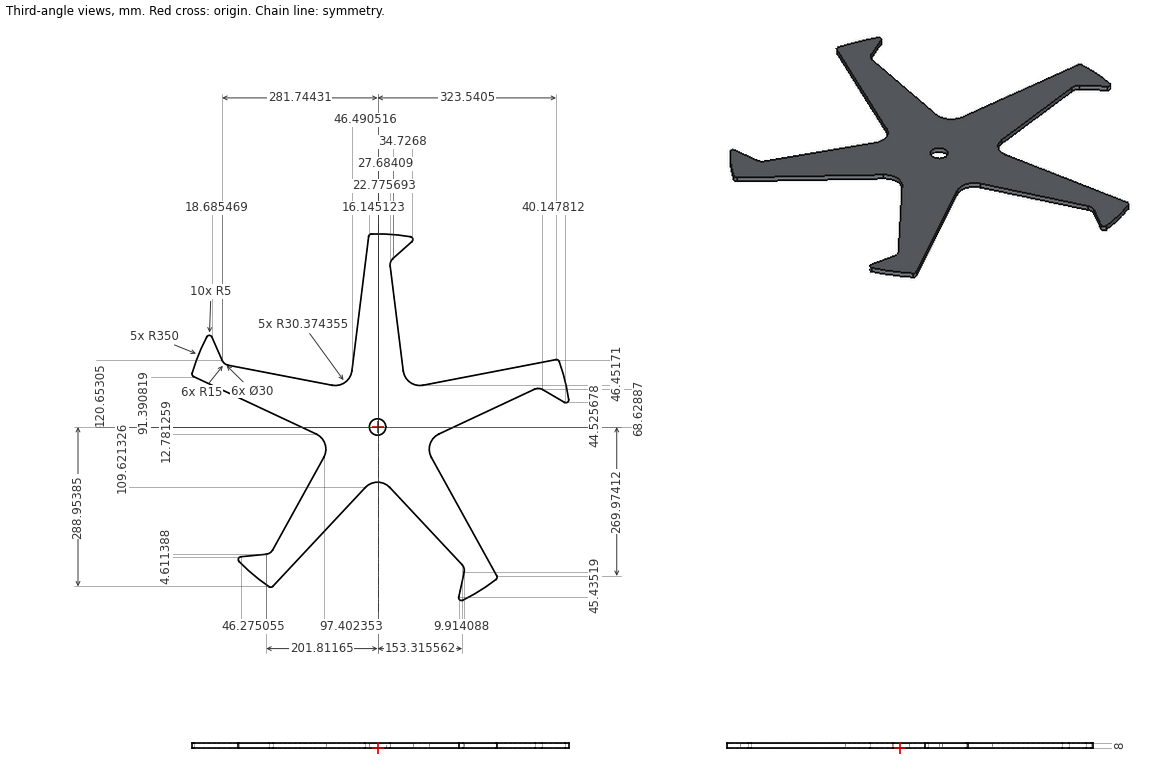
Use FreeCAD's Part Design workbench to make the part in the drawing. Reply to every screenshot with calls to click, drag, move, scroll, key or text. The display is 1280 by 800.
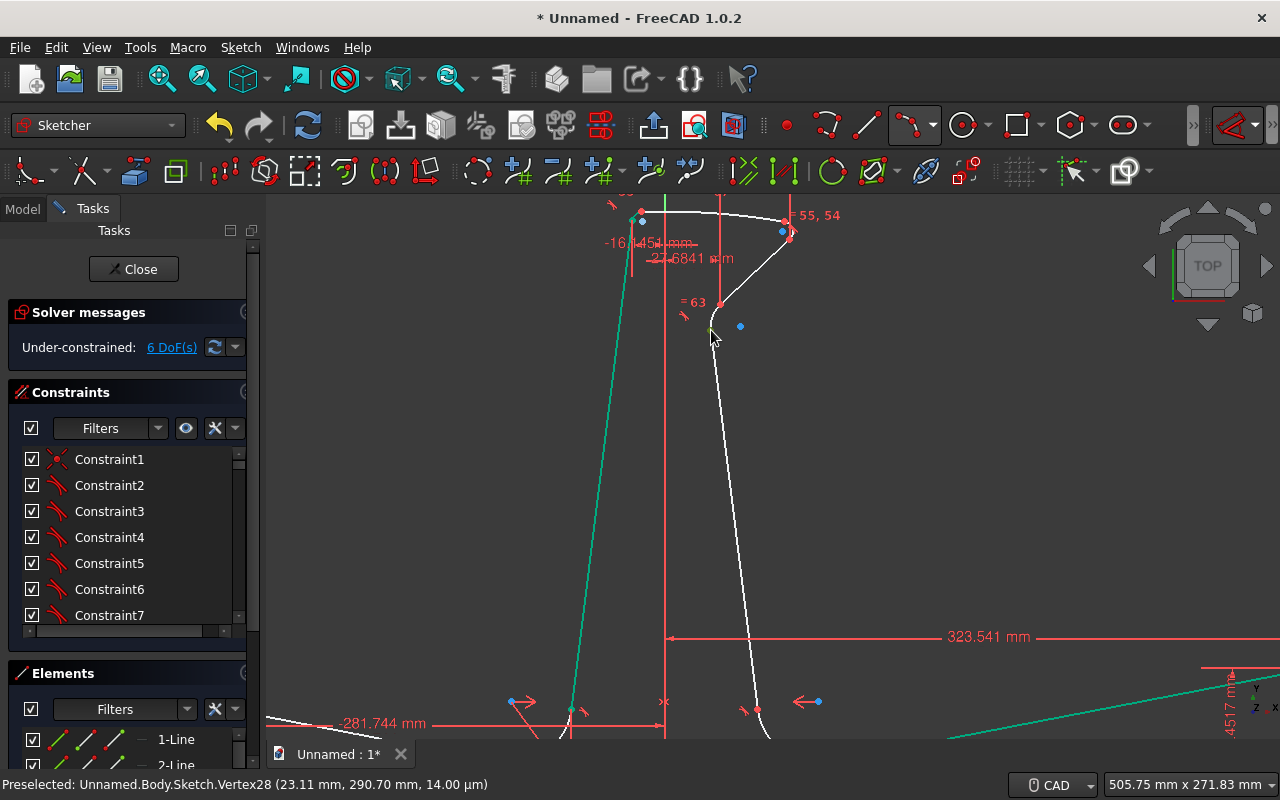
key(l)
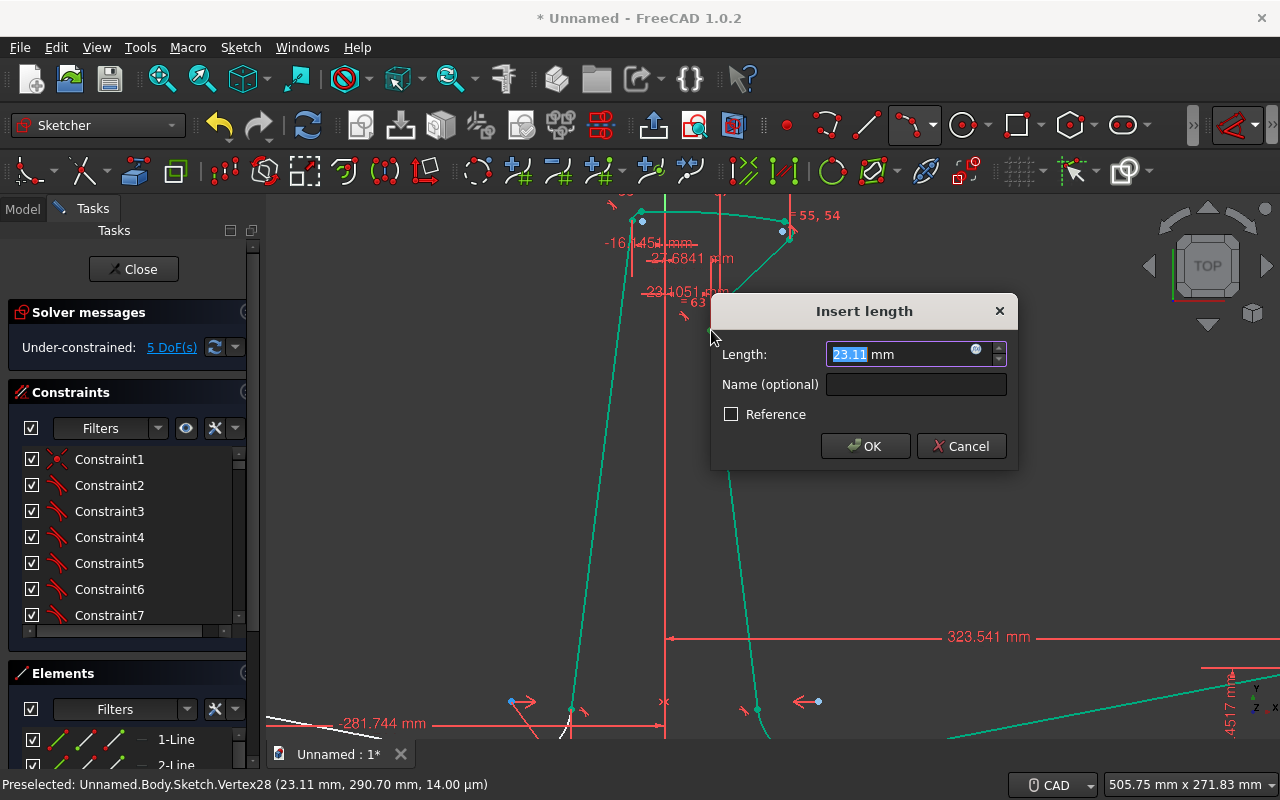
text(22.775693)
key(Return)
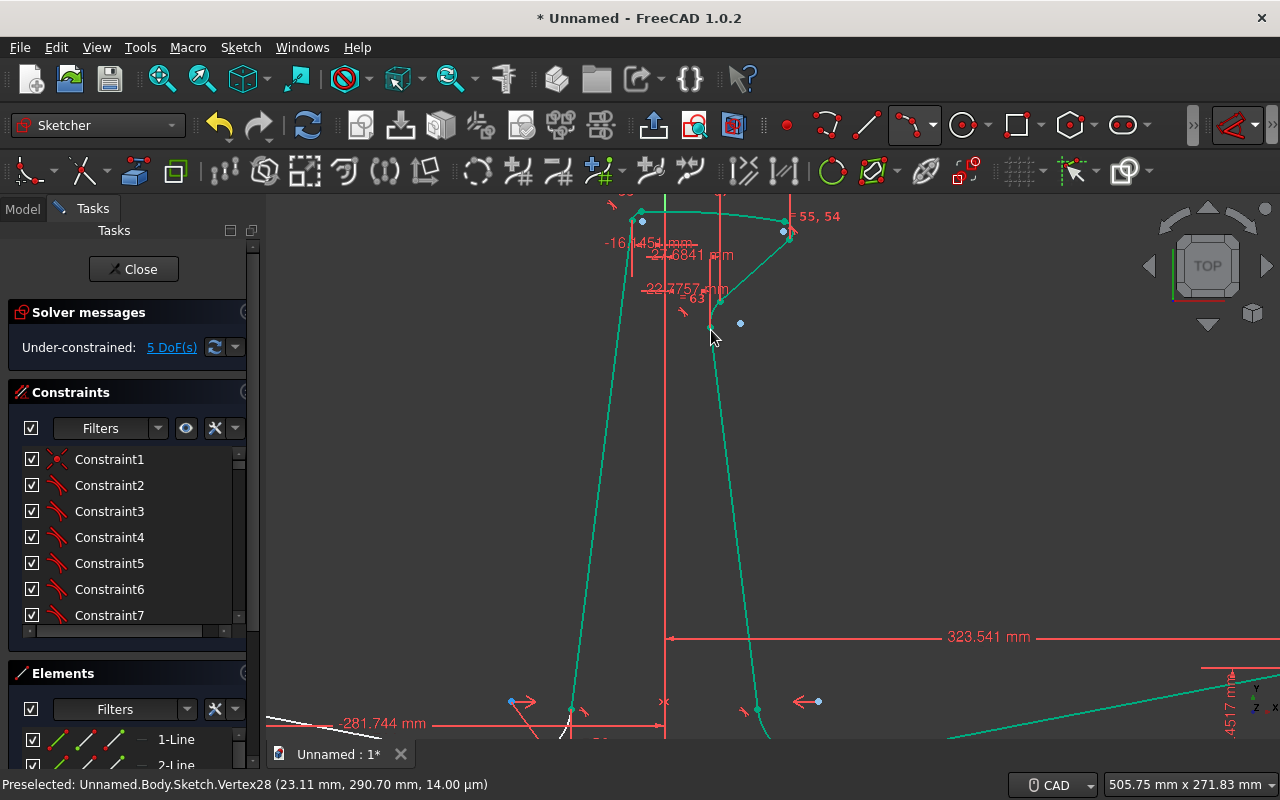
scroll(714, 332, down, 7)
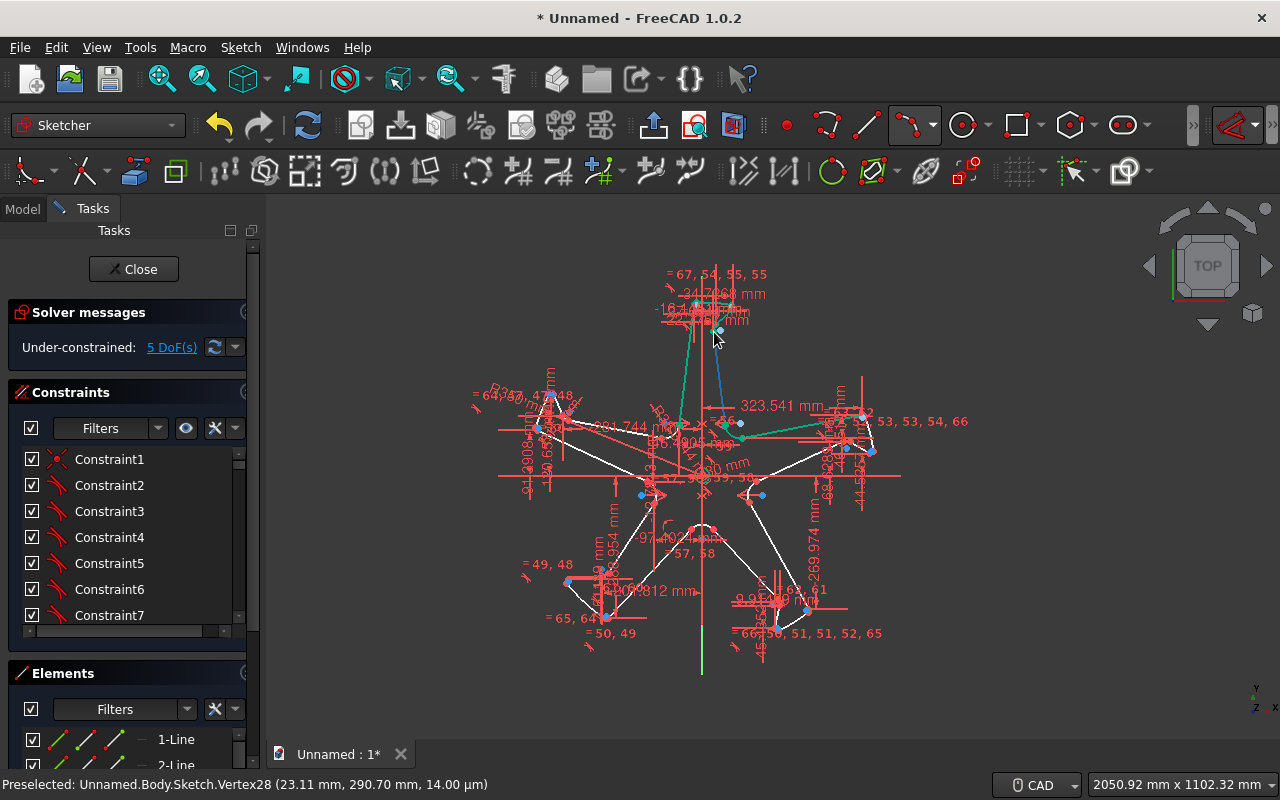
scroll(560, 410, up, 8)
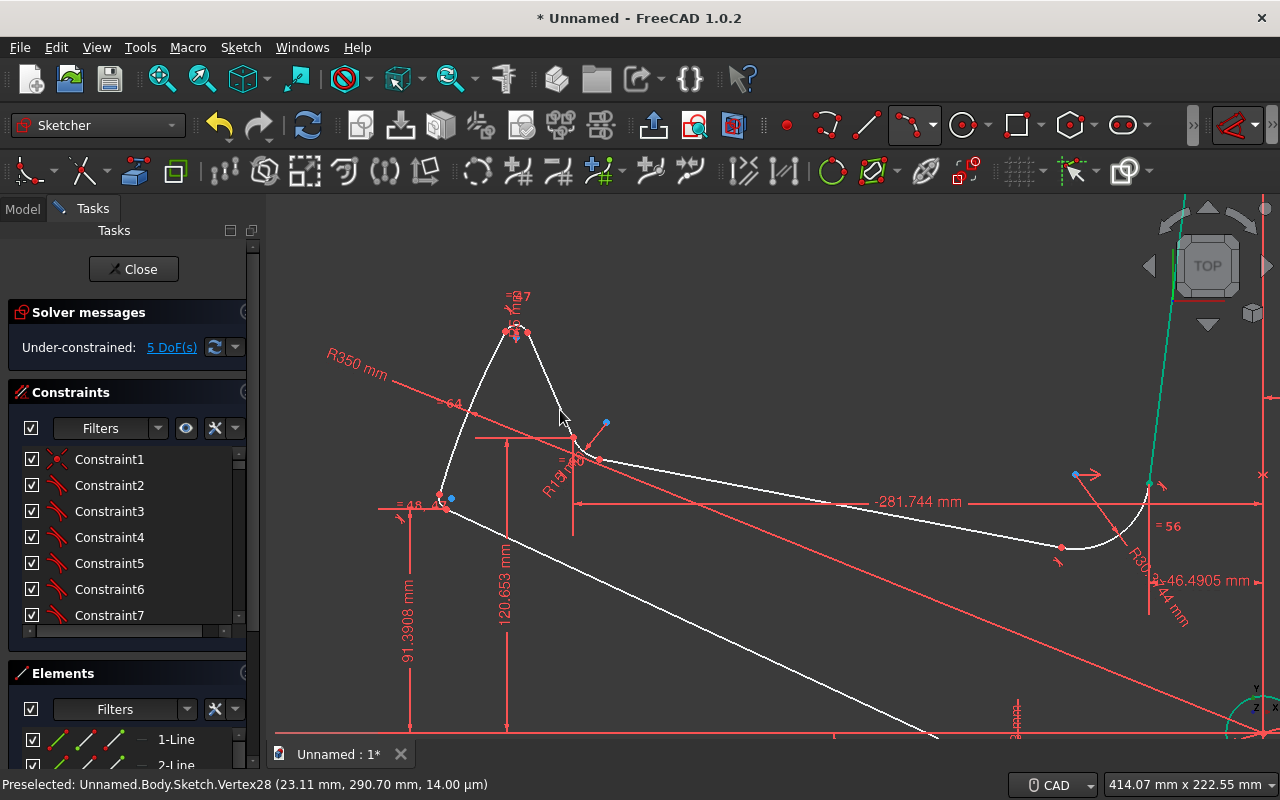
click(559, 406)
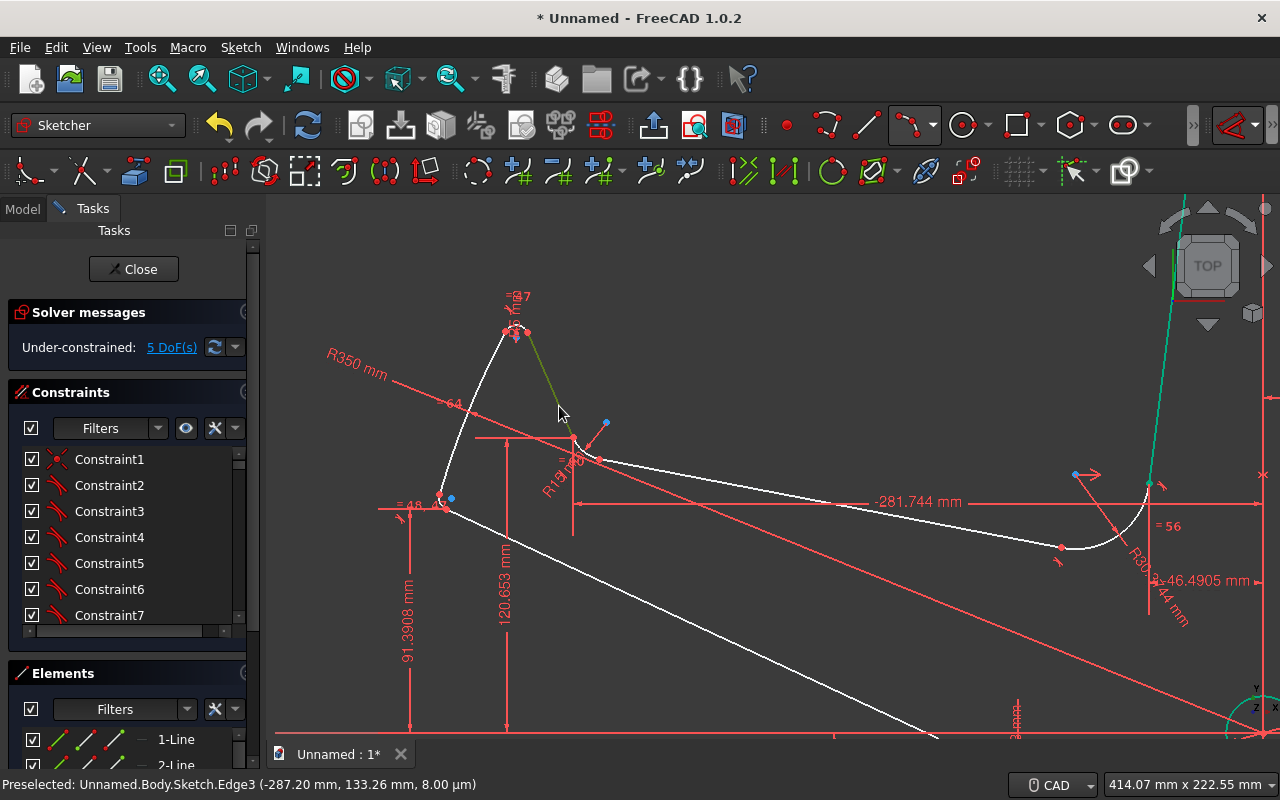
key(l)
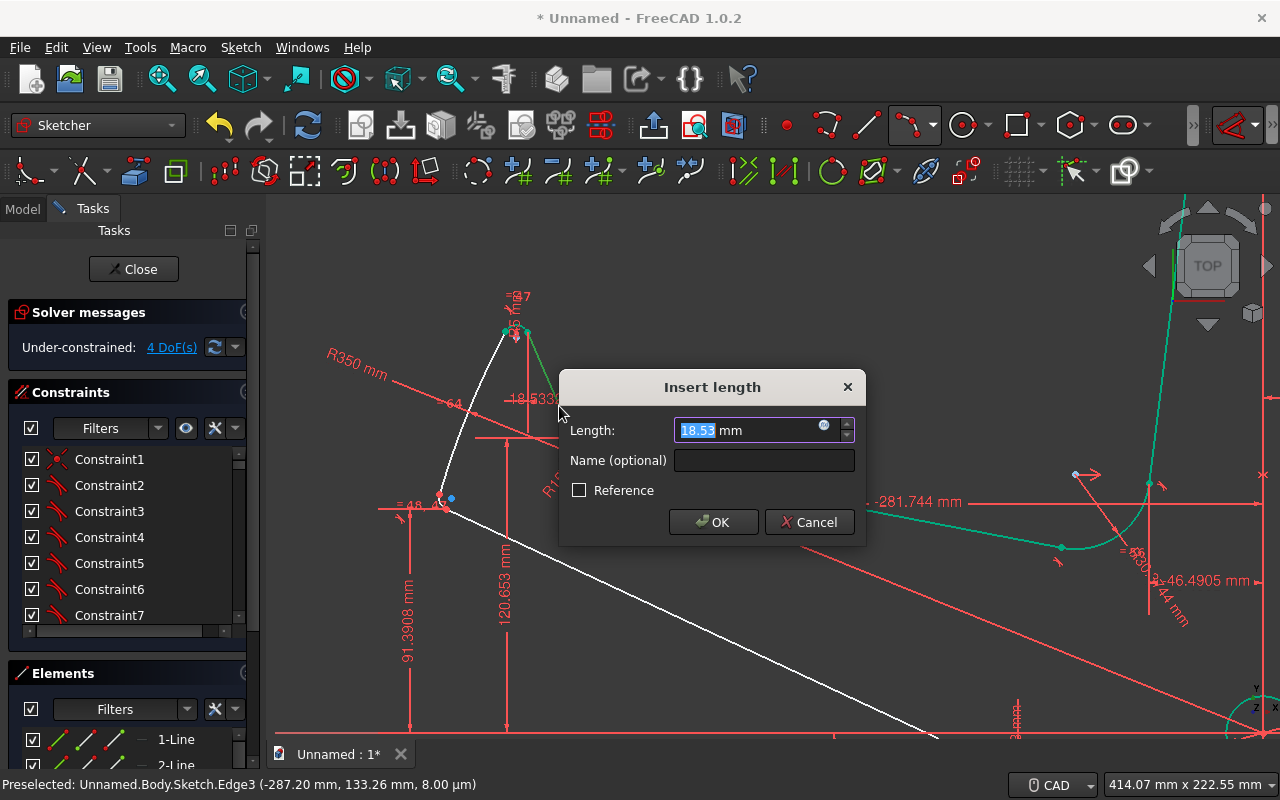
text(18.685469)
key(Return)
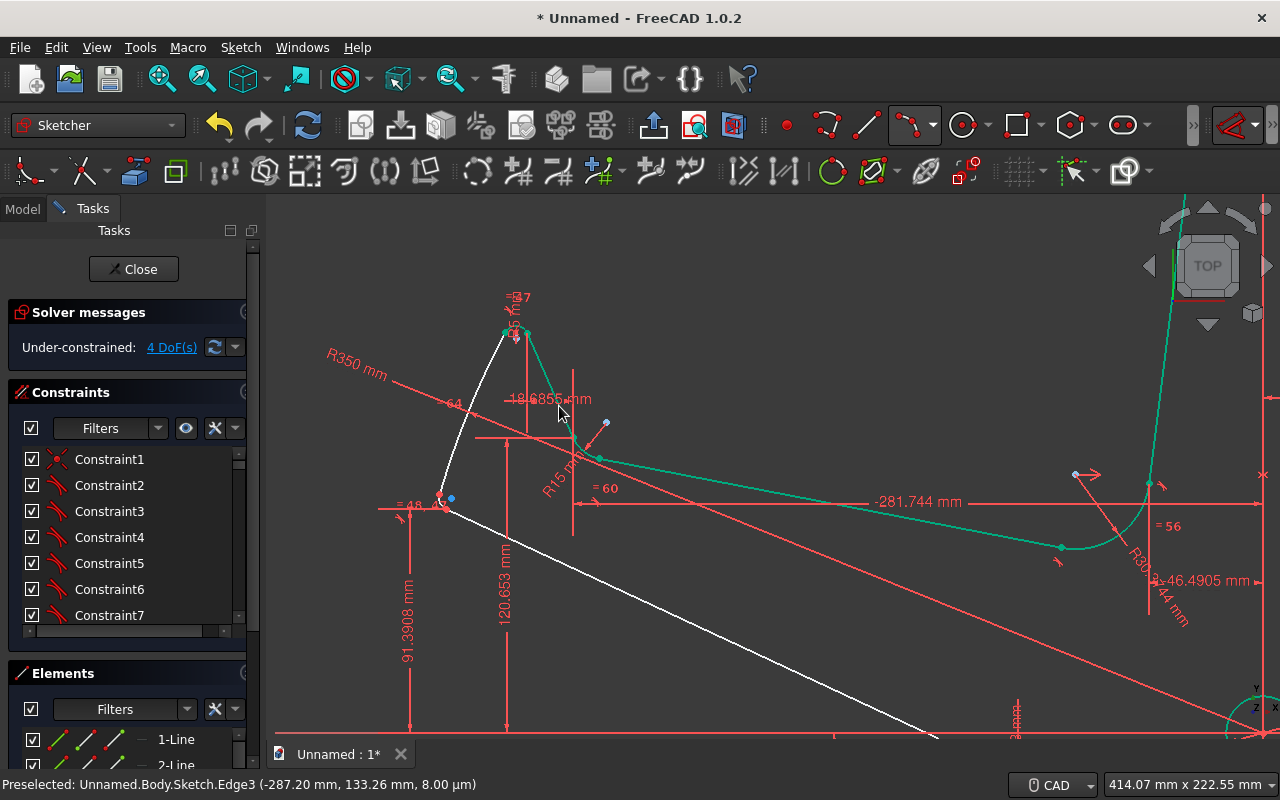
scroll(560, 410, down, 8)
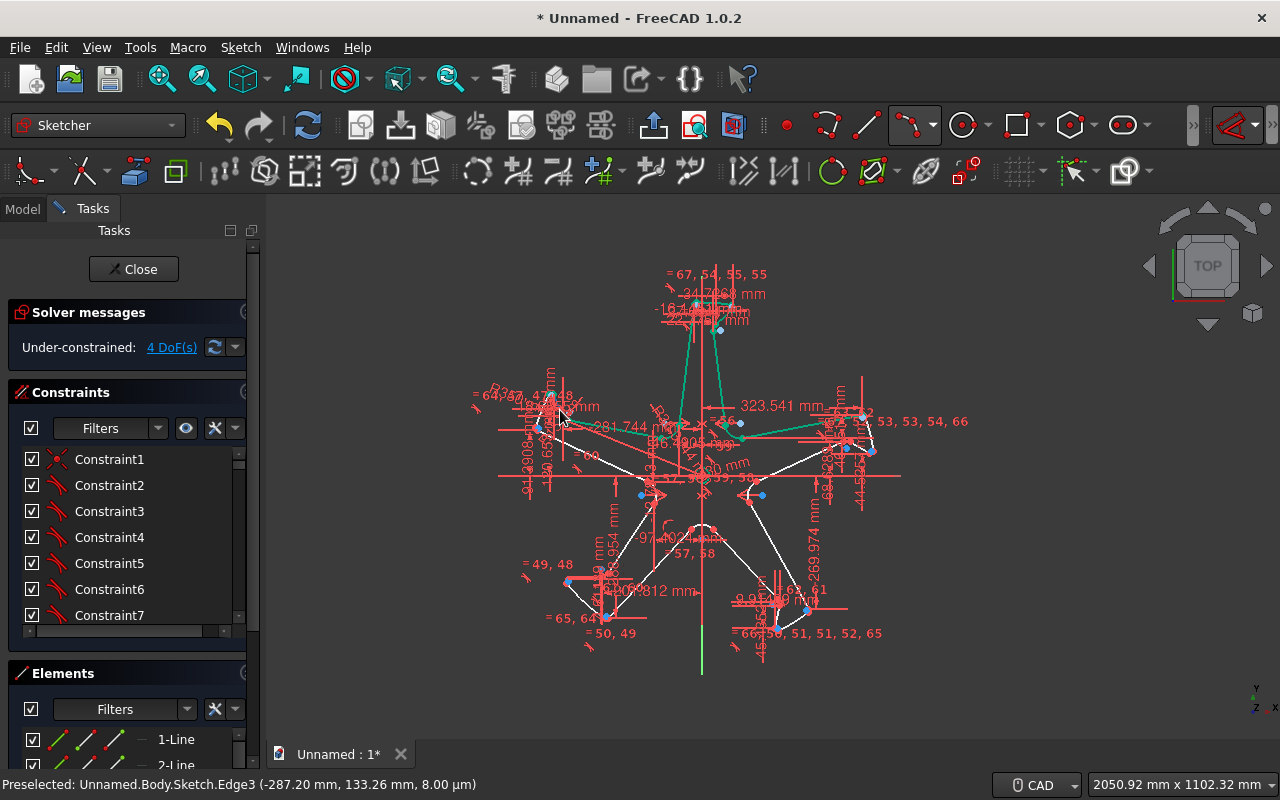
scroll(592, 577, up, 3)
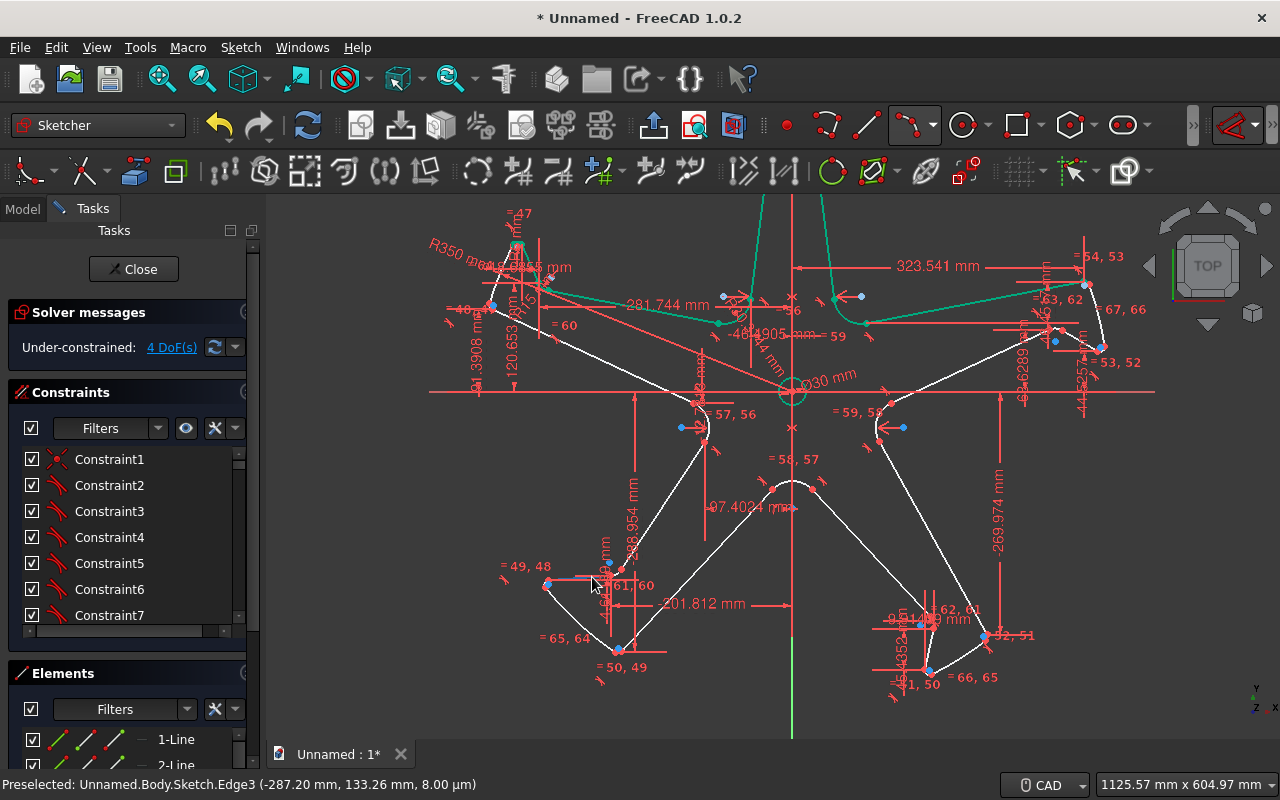
click(592, 577)